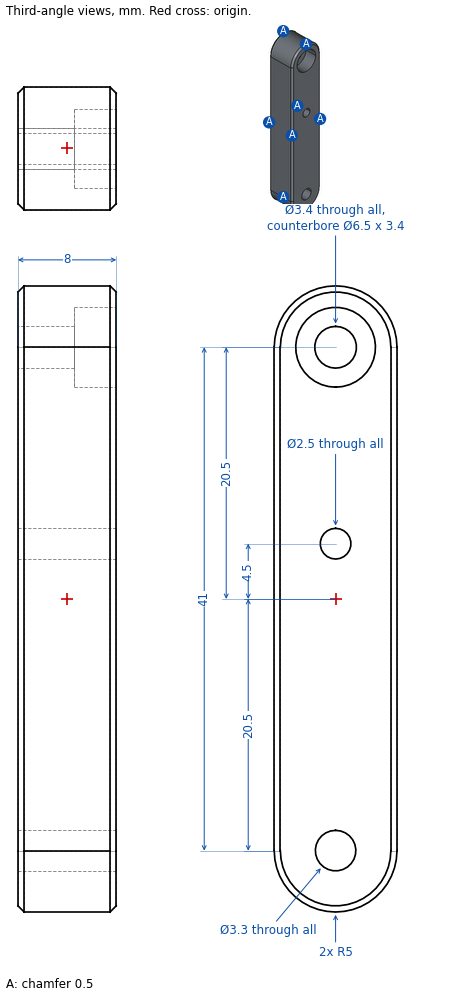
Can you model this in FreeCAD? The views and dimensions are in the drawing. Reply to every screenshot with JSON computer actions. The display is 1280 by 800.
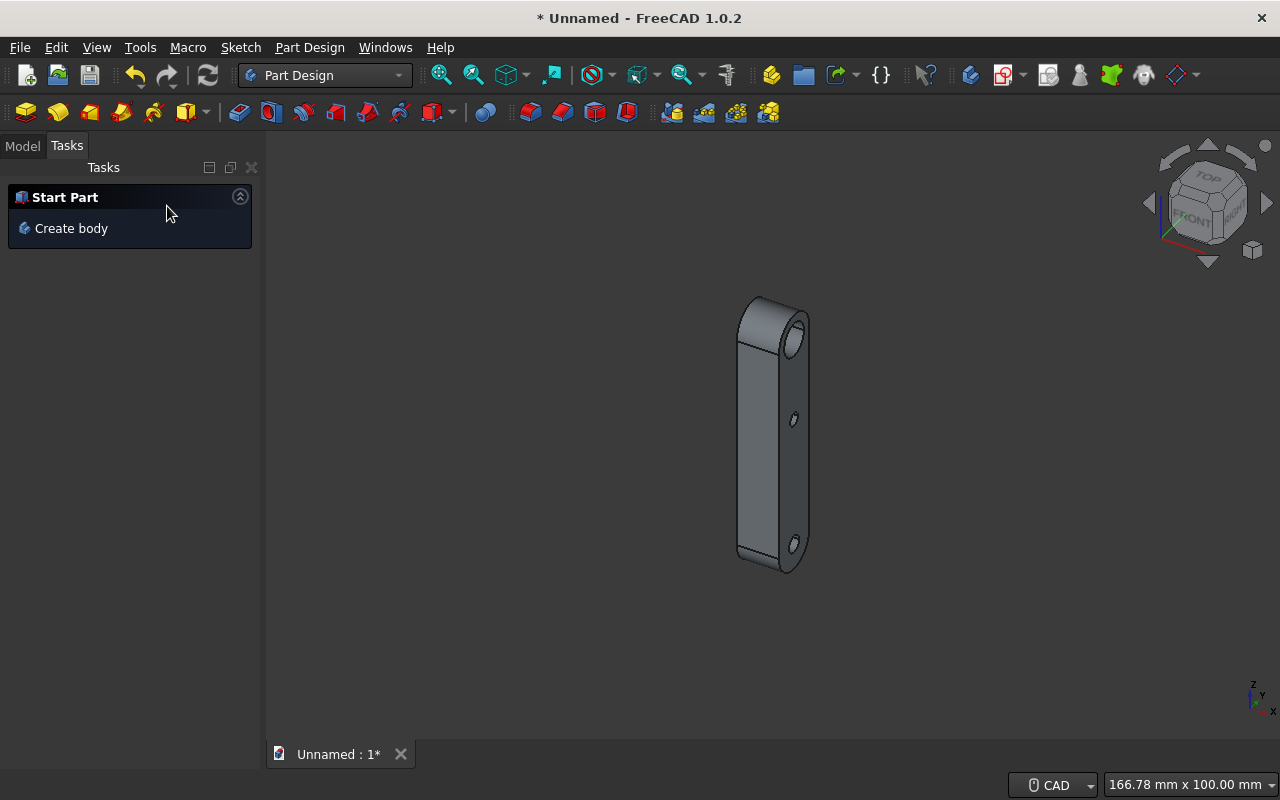
{"action": "left_click", "coordinate": [794, 314]}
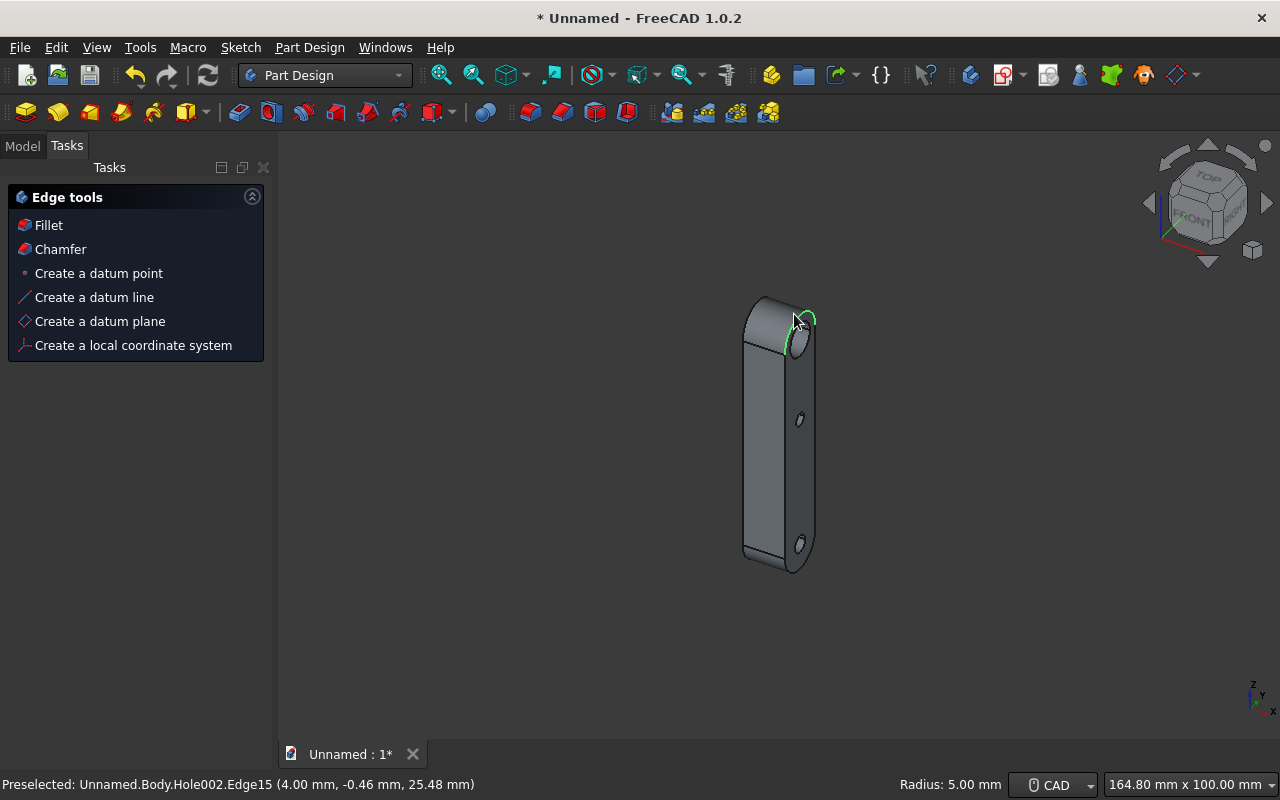
{"action": "left_click", "coordinate": [785, 456], "text": "ctrl"}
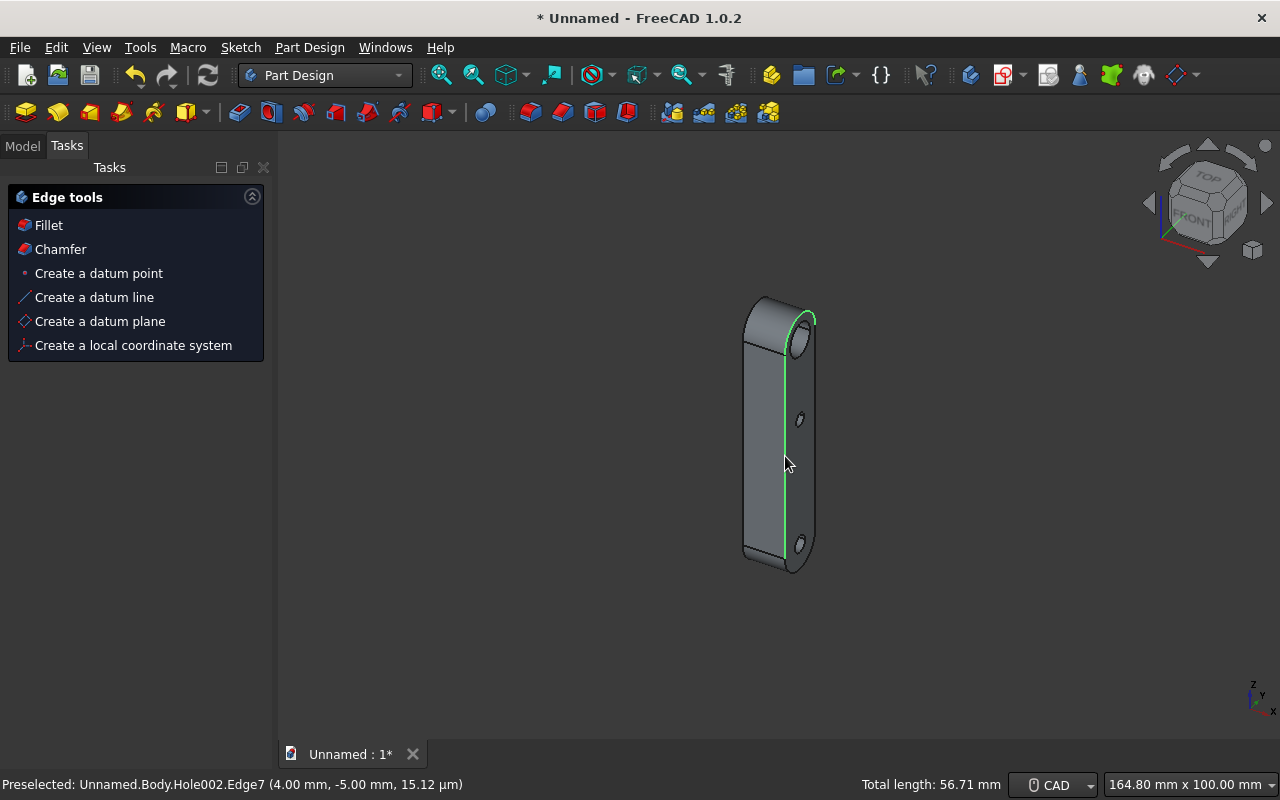
{"action": "left_click", "coordinate": [791, 572], "text": "ctrl"}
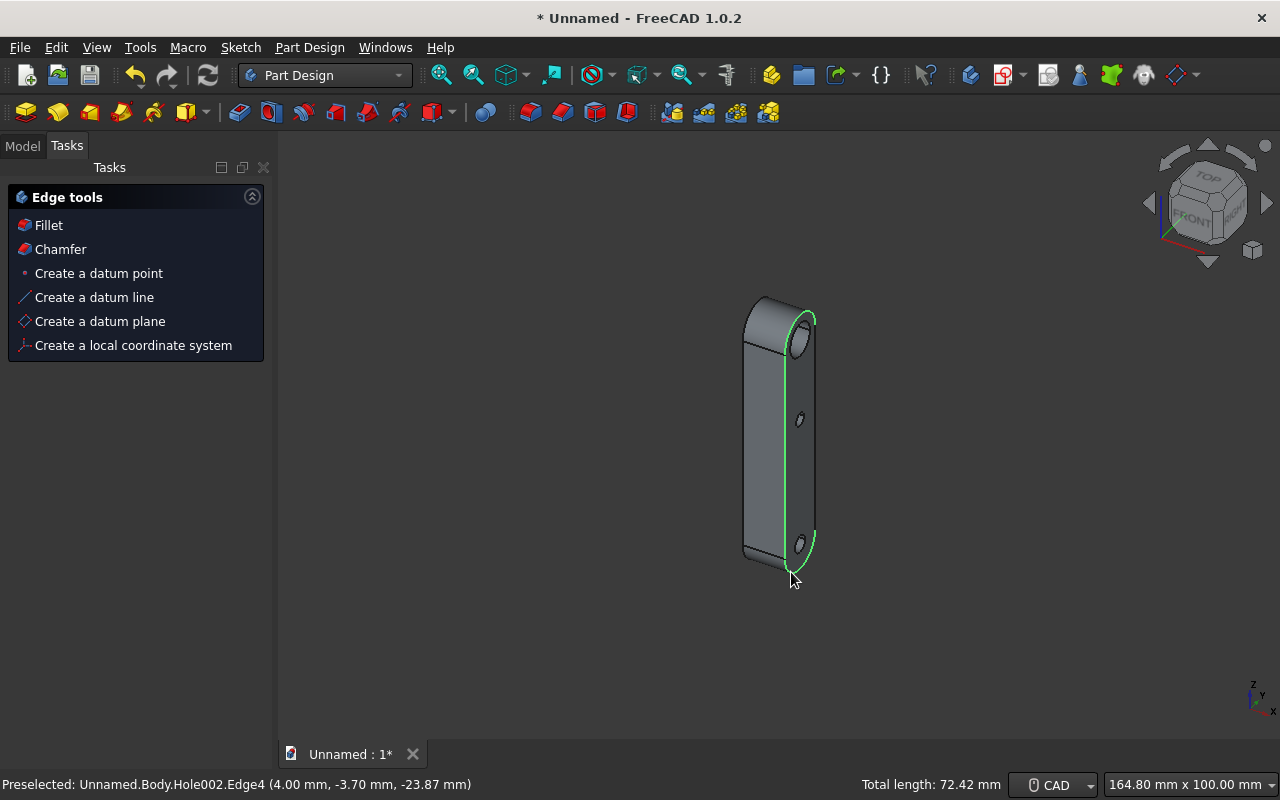
{"action": "left_click", "coordinate": [758, 300], "text": "ctrl"}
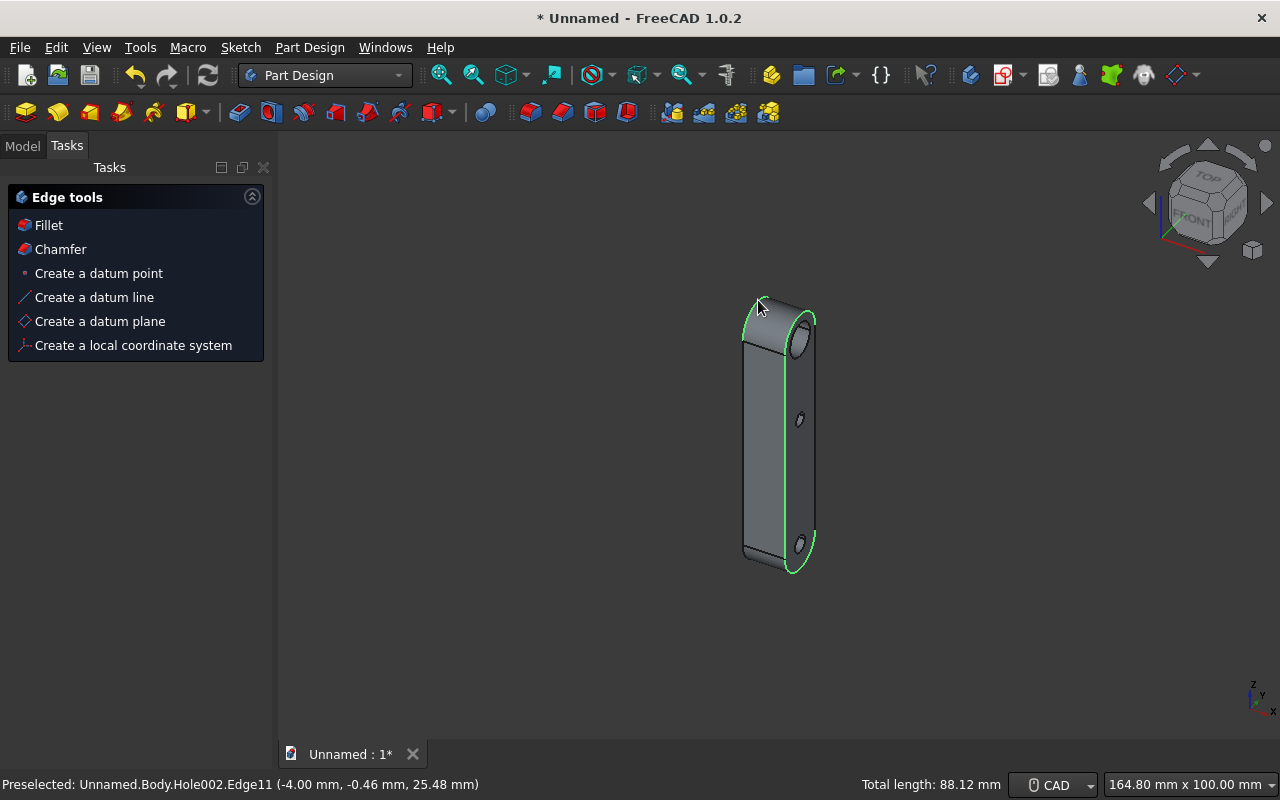
{"action": "left_click", "coordinate": [744, 552], "text": "ctrl"}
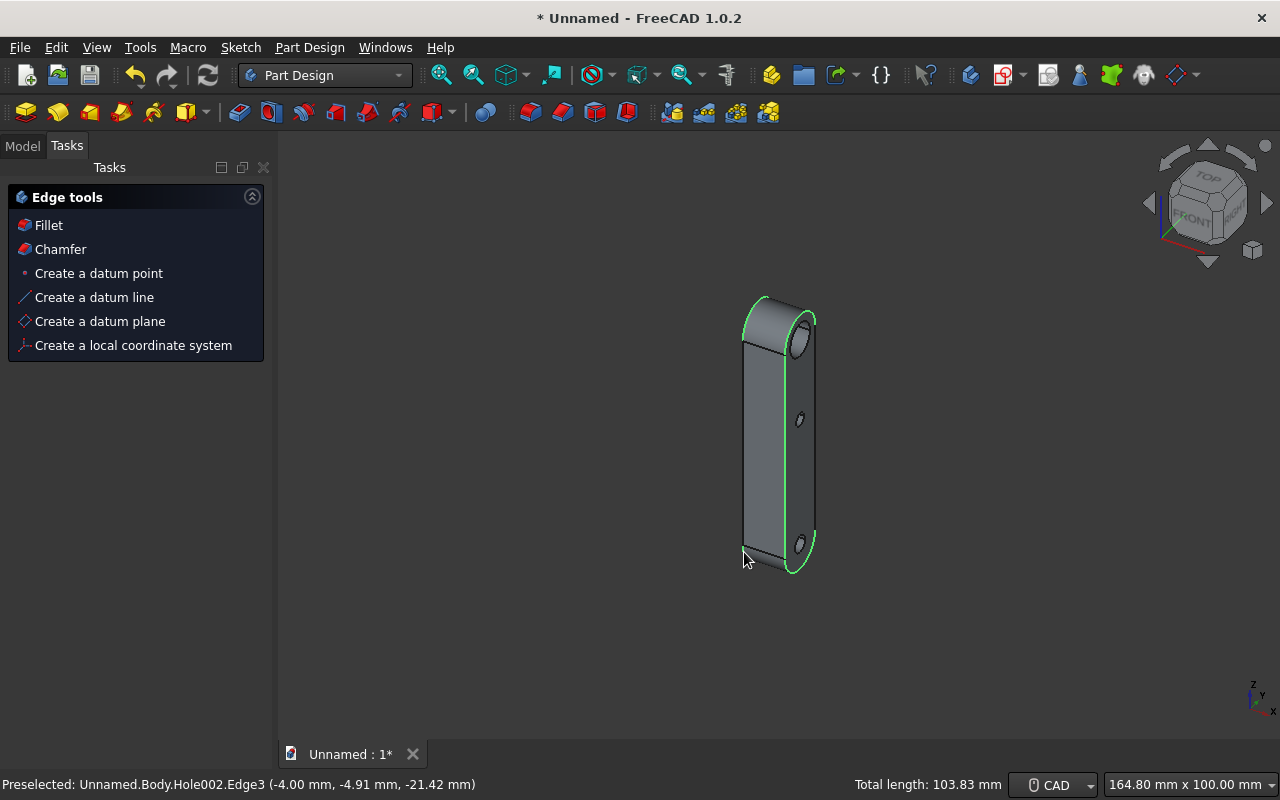
{"action": "key", "text": "0"}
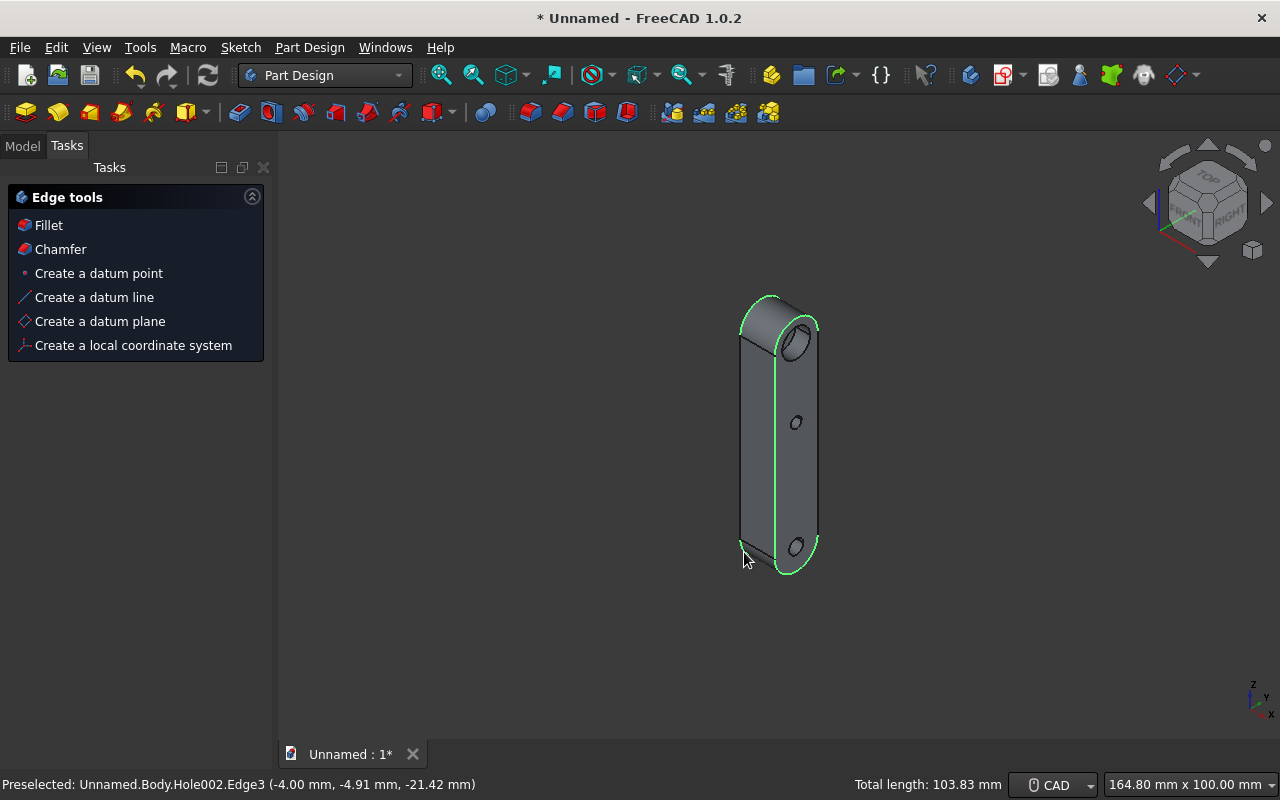
{"action": "key", "text": "2"}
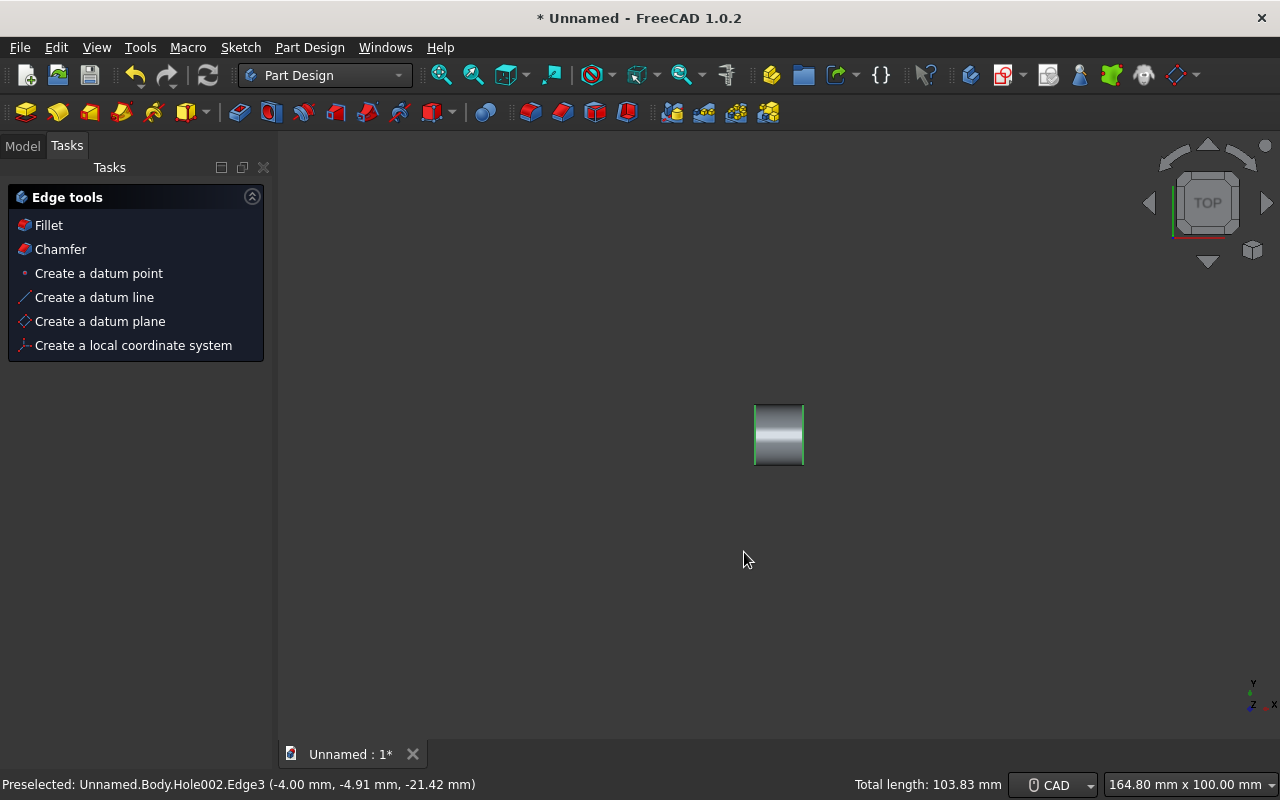
{"action": "key", "text": "v f"}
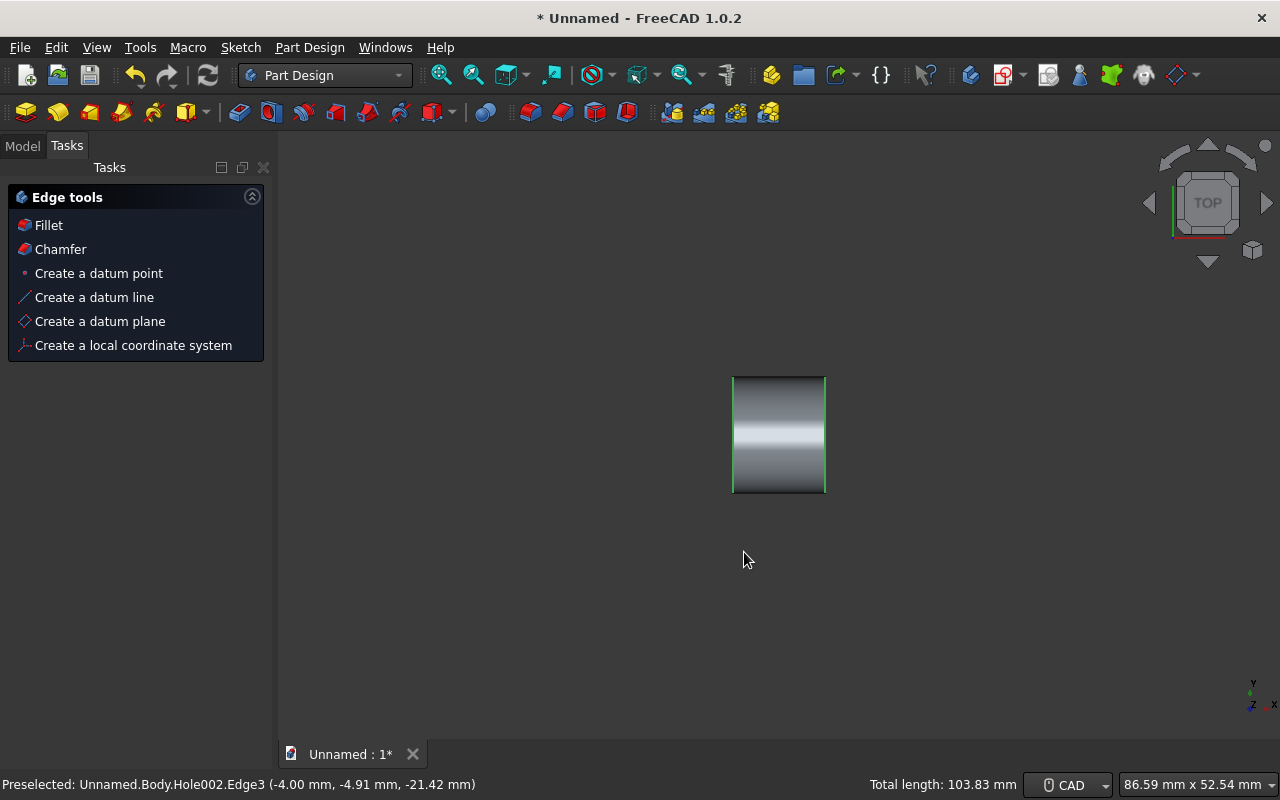
{"action": "key", "text": "1"}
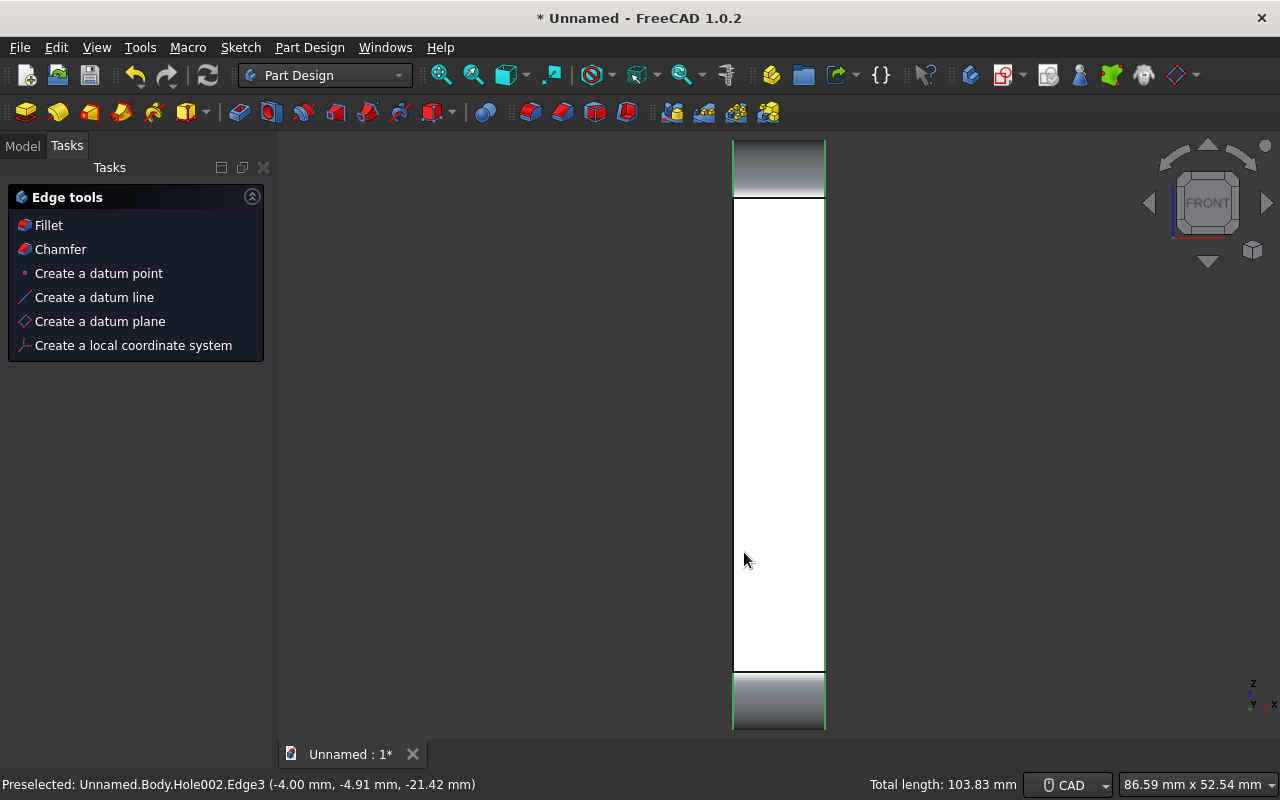
{"action": "left_click", "coordinate": [733, 434], "text": "ctrl"}